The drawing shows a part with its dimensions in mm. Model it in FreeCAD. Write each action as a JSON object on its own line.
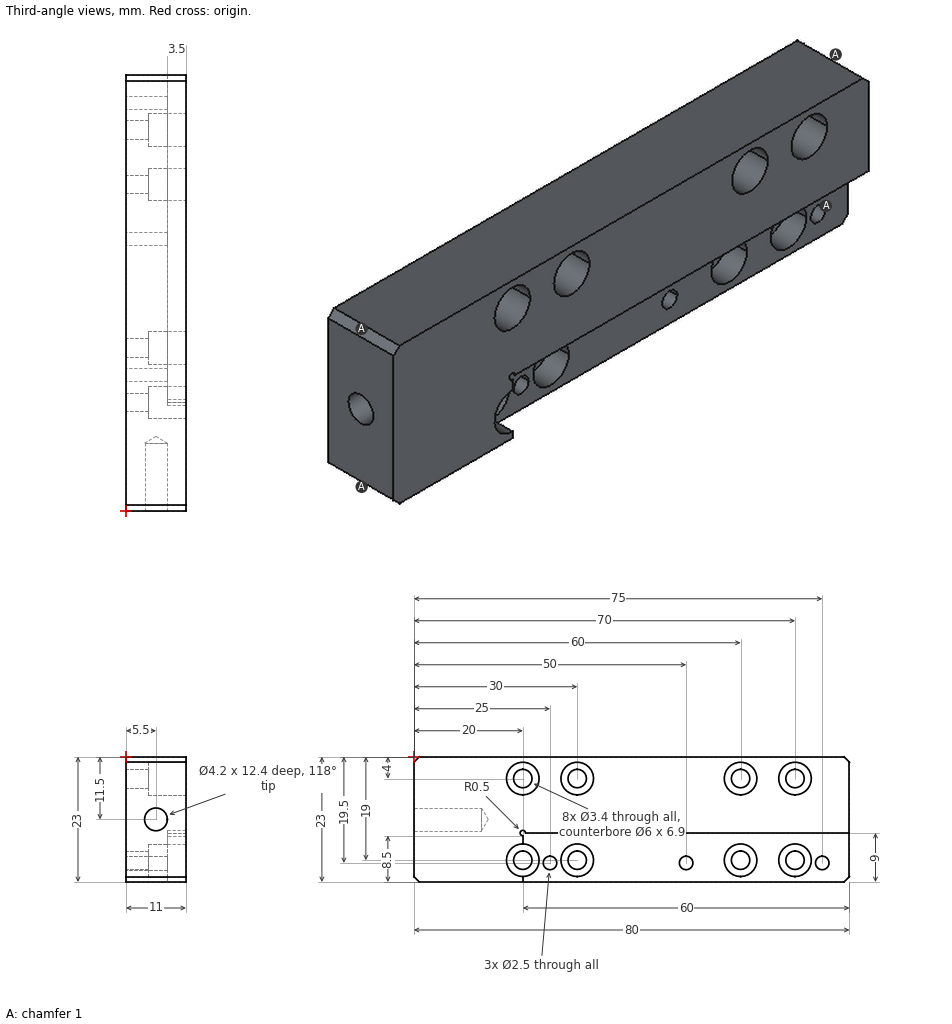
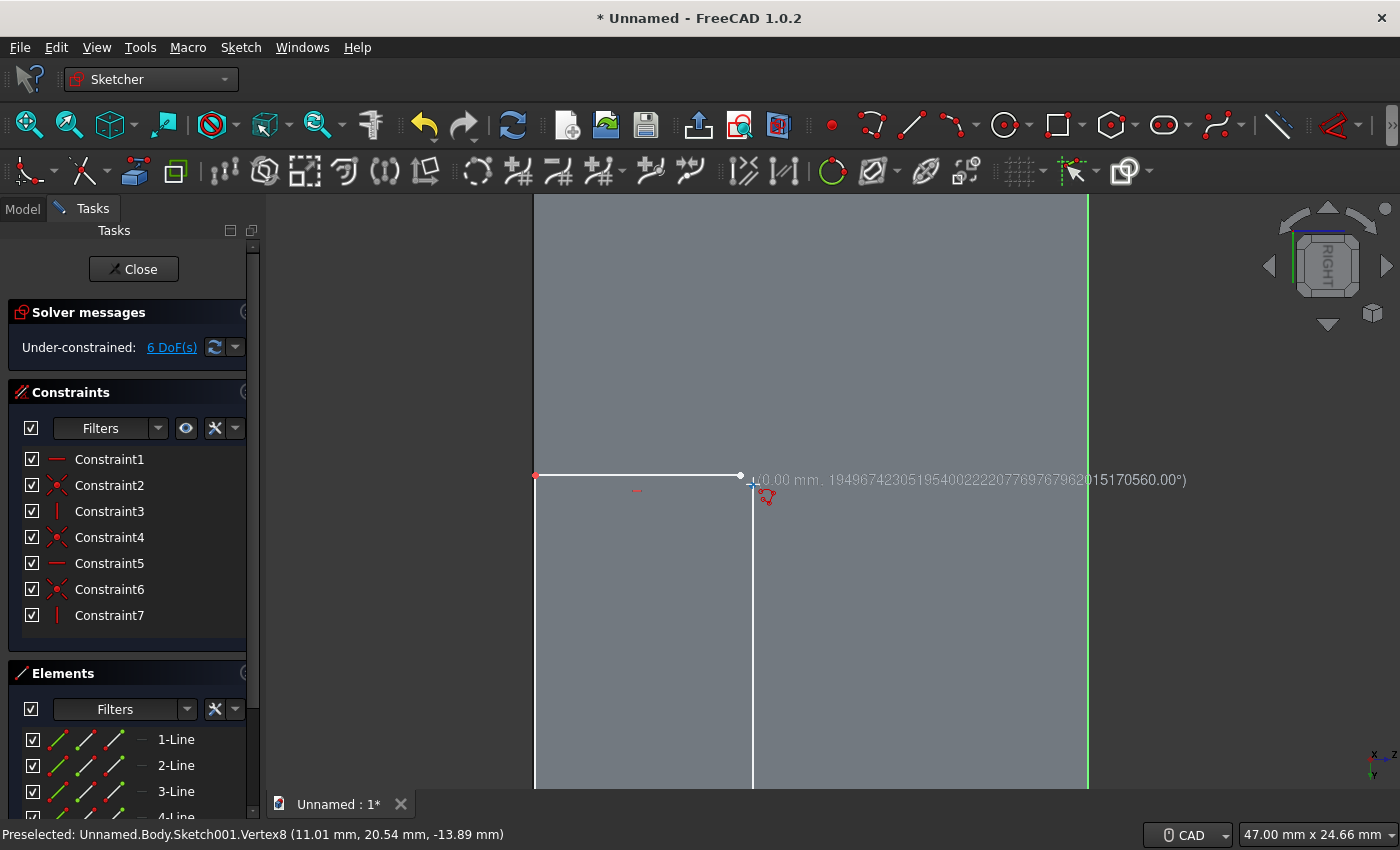
{"action": "left_click", "coordinate": [952, 126]}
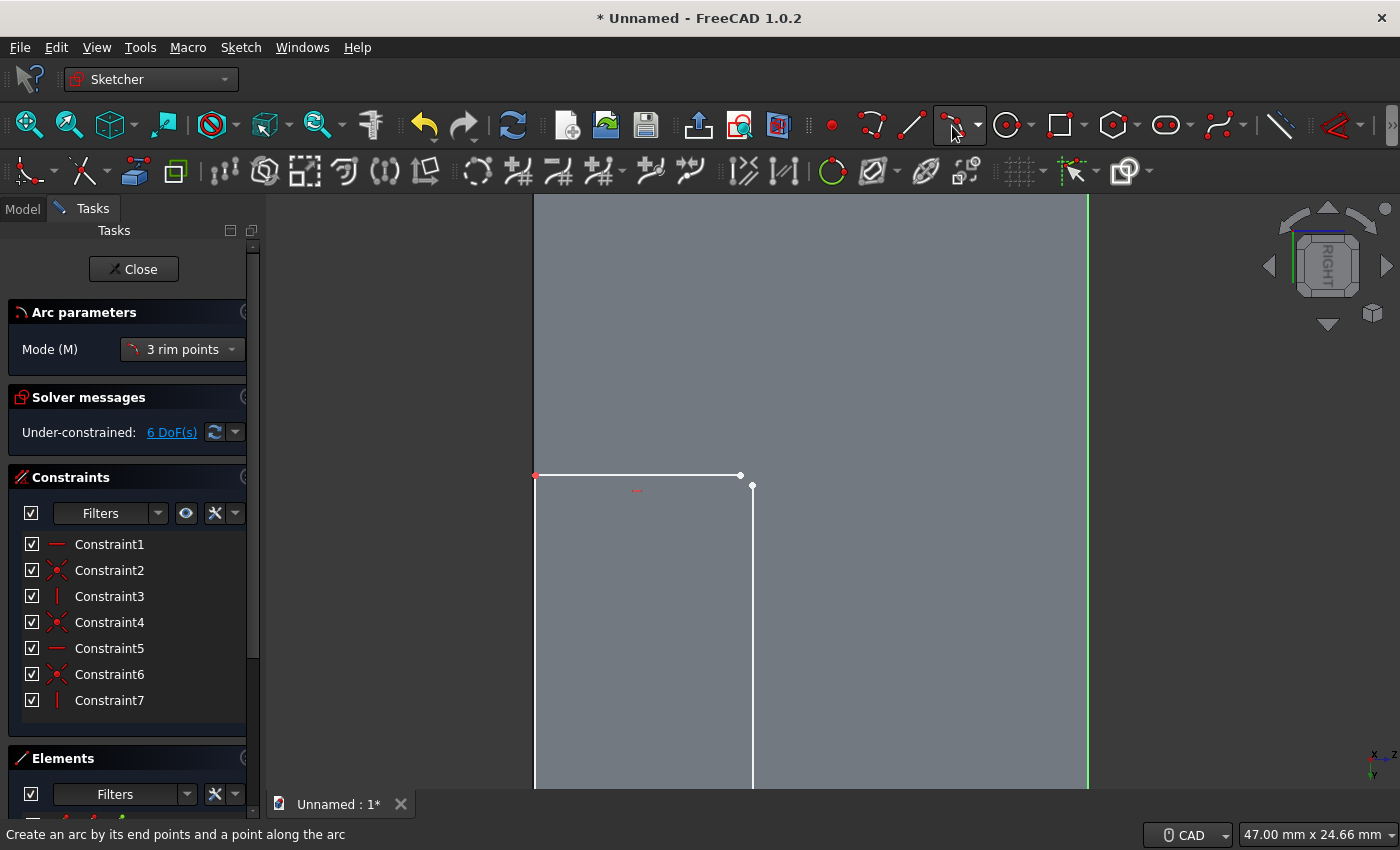
{"action": "left_click", "coordinate": [753, 485]}
{"action": "left_click", "coordinate": [741, 475]}
{"action": "left_click", "coordinate": [759, 464]}
{"action": "key", "text": "Escape"}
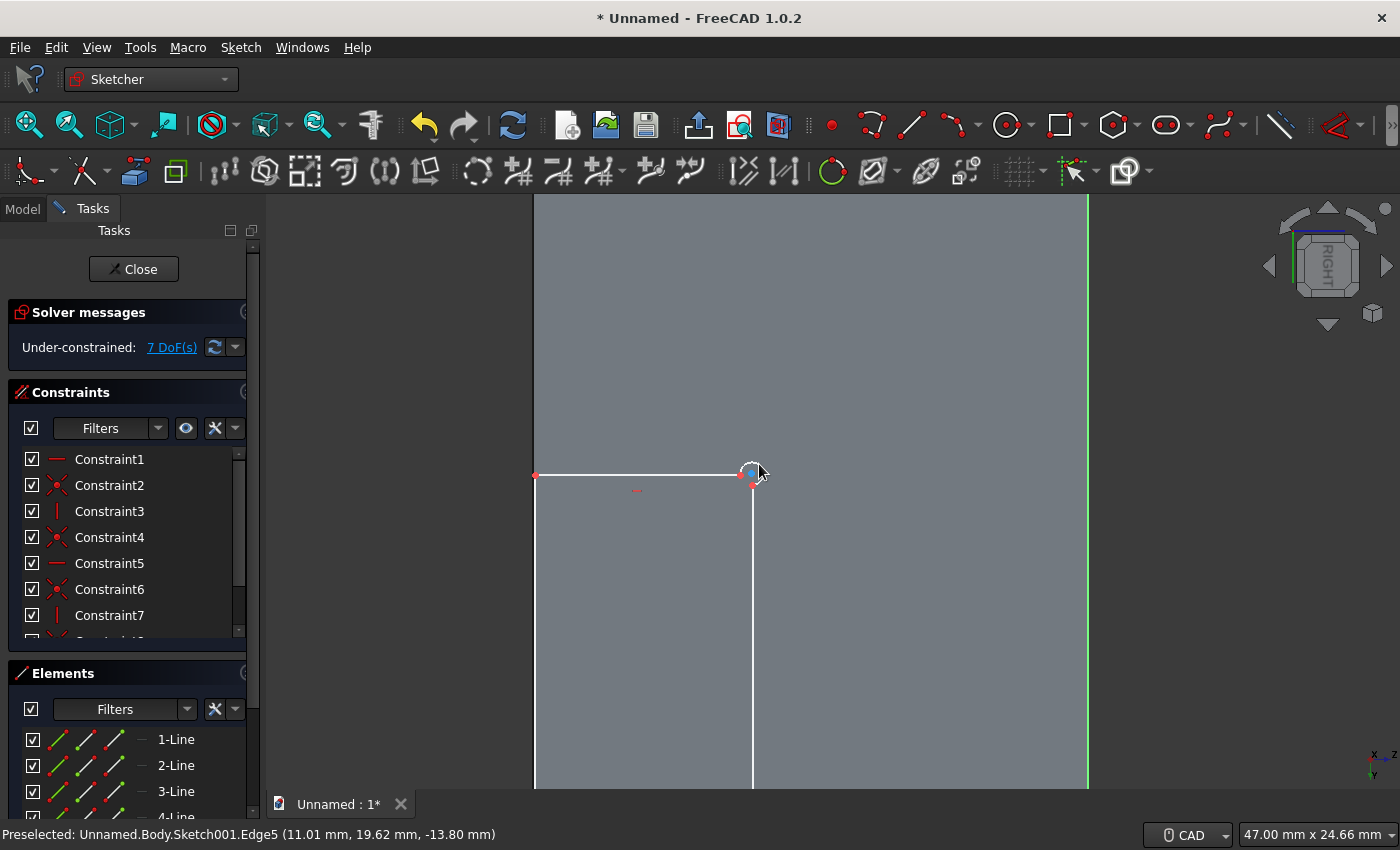
{"action": "left_click", "coordinate": [1336, 126]}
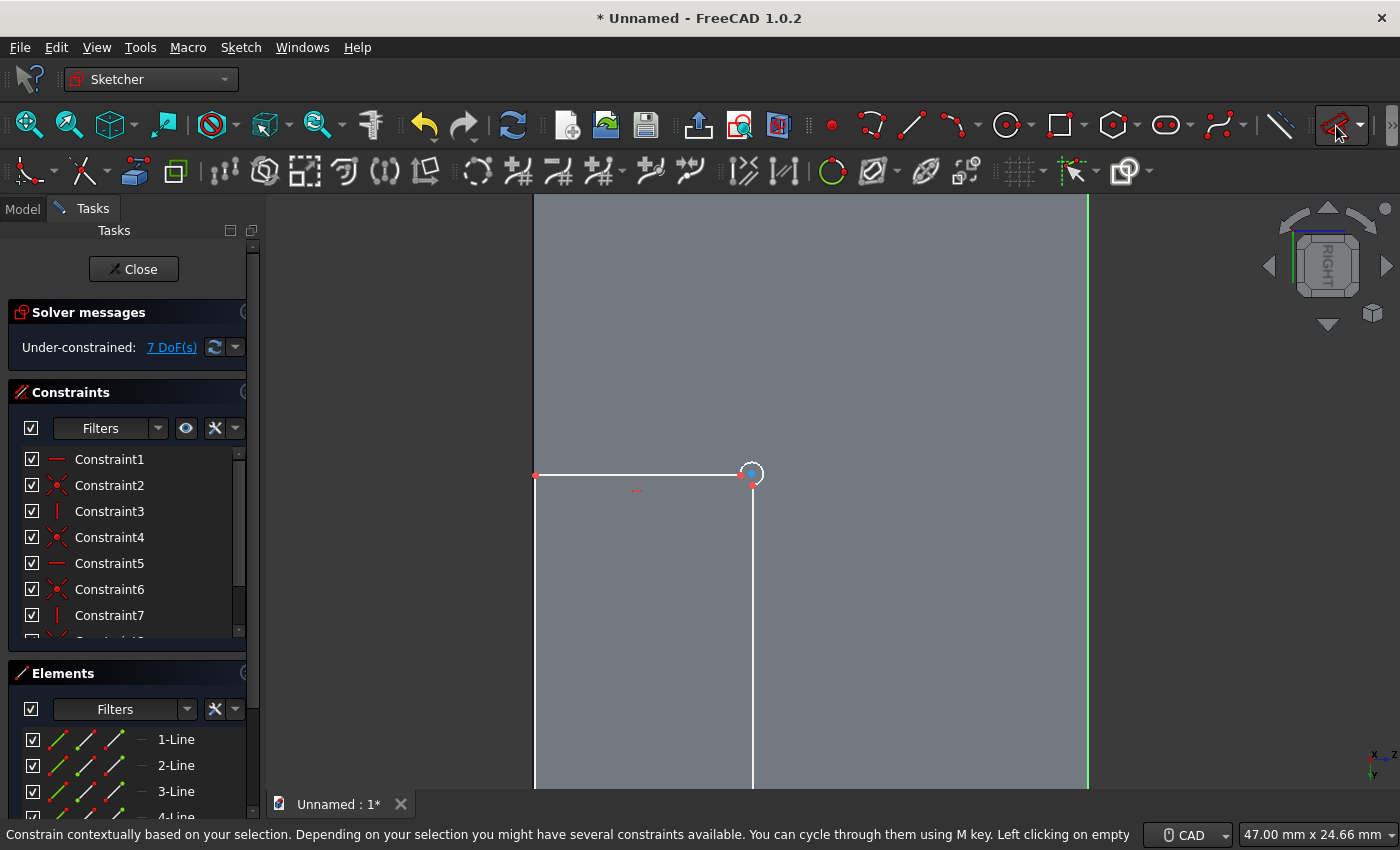
{"action": "scroll", "coordinate": [763, 474], "scroll_direction": "up", "scroll_amount": 6}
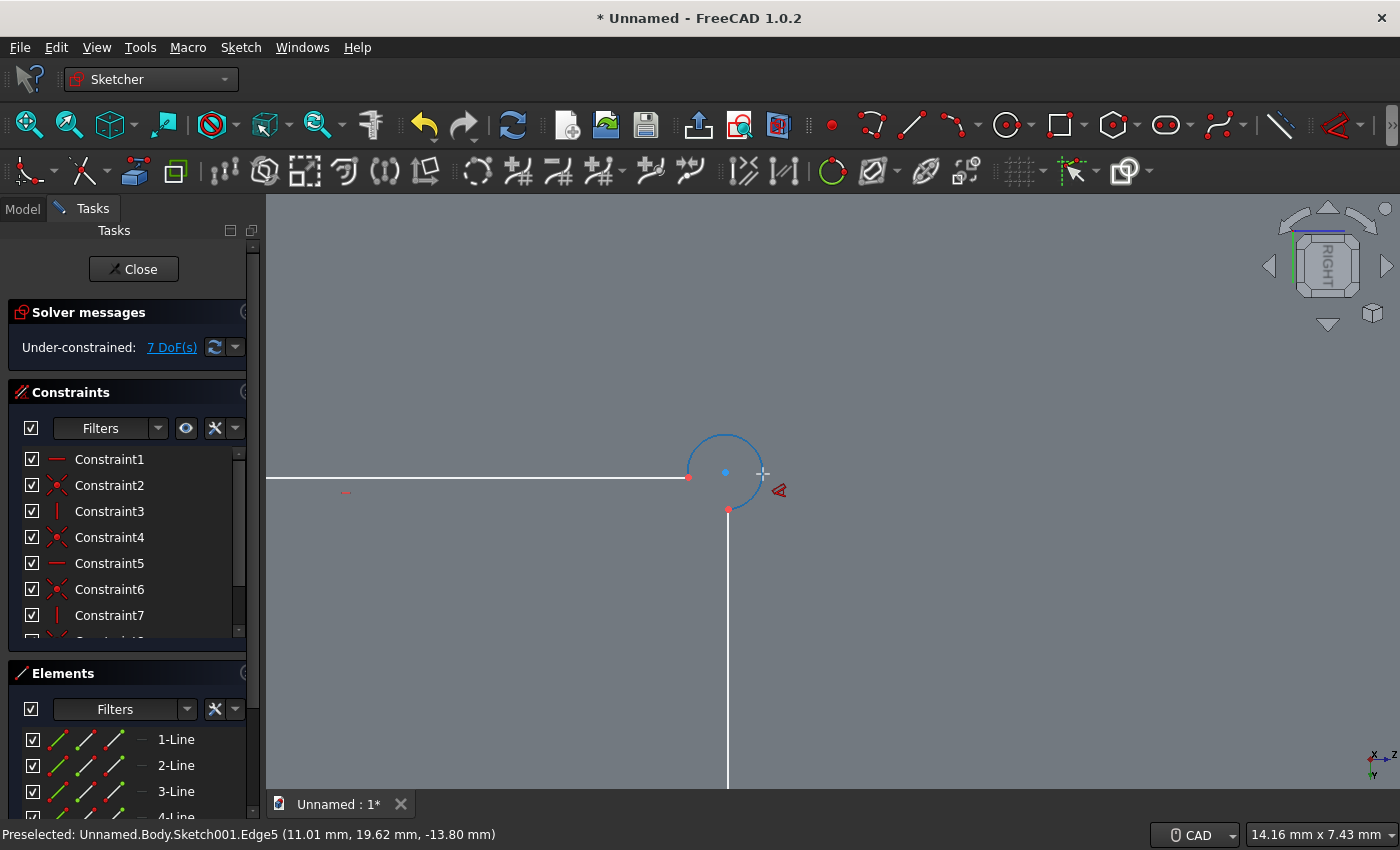
{"action": "left_click", "coordinate": [762, 474]}
{"action": "left_click", "coordinate": [794, 476]}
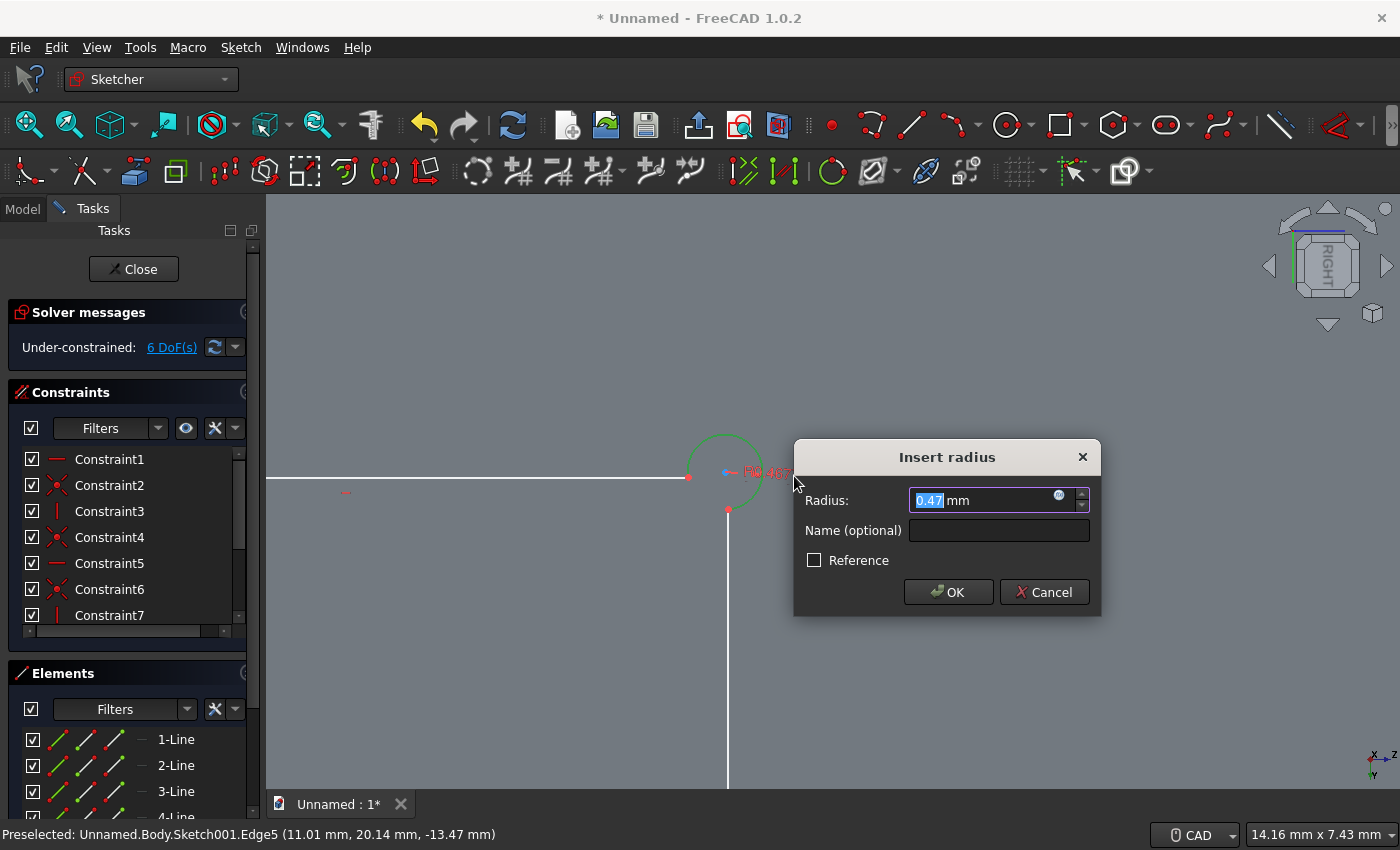
{"action": "type", "text": "0.5"}
{"action": "key", "text": "Return"}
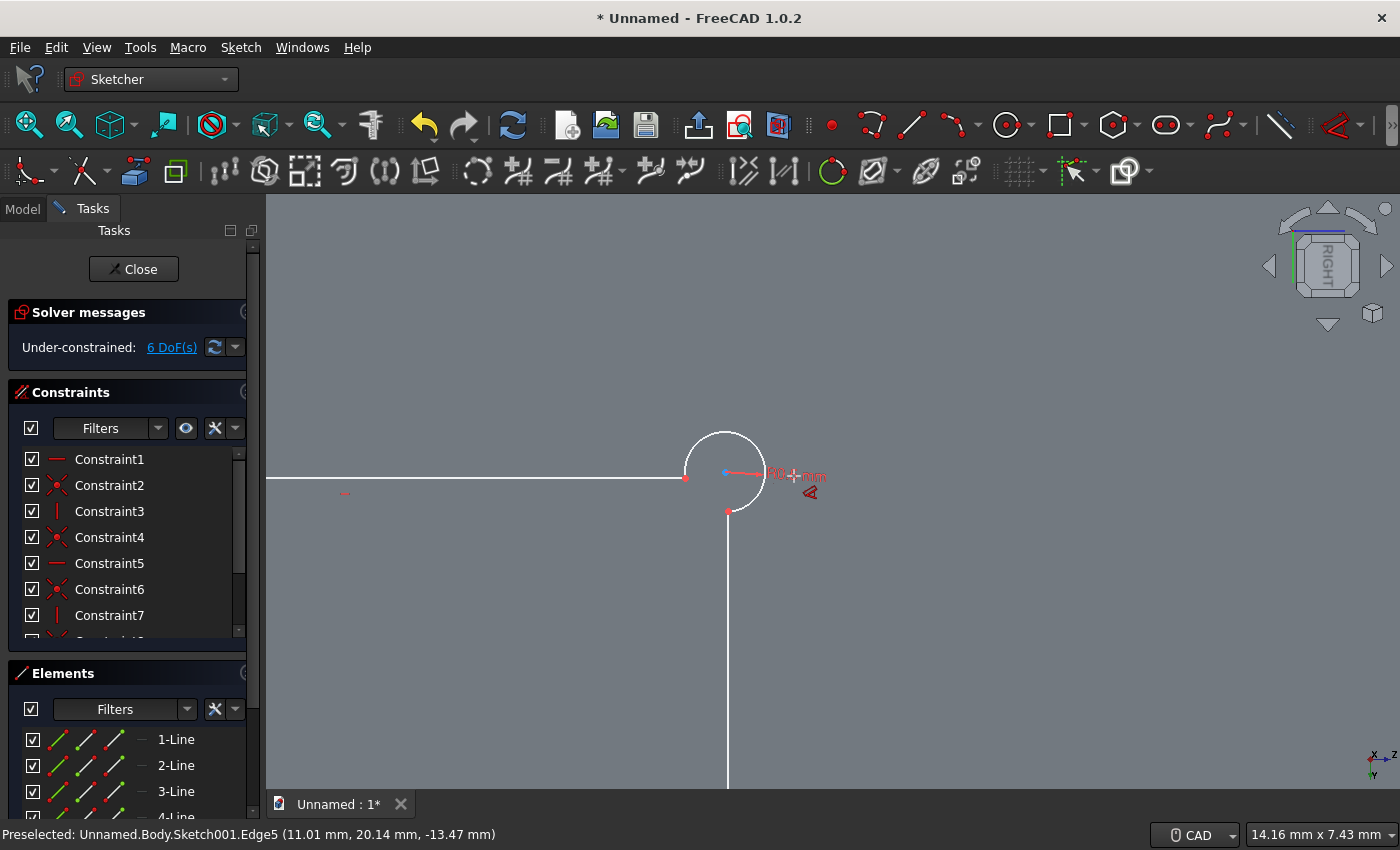
{"action": "scroll", "coordinate": [754, 389], "scroll_direction": "down", "scroll_amount": 14}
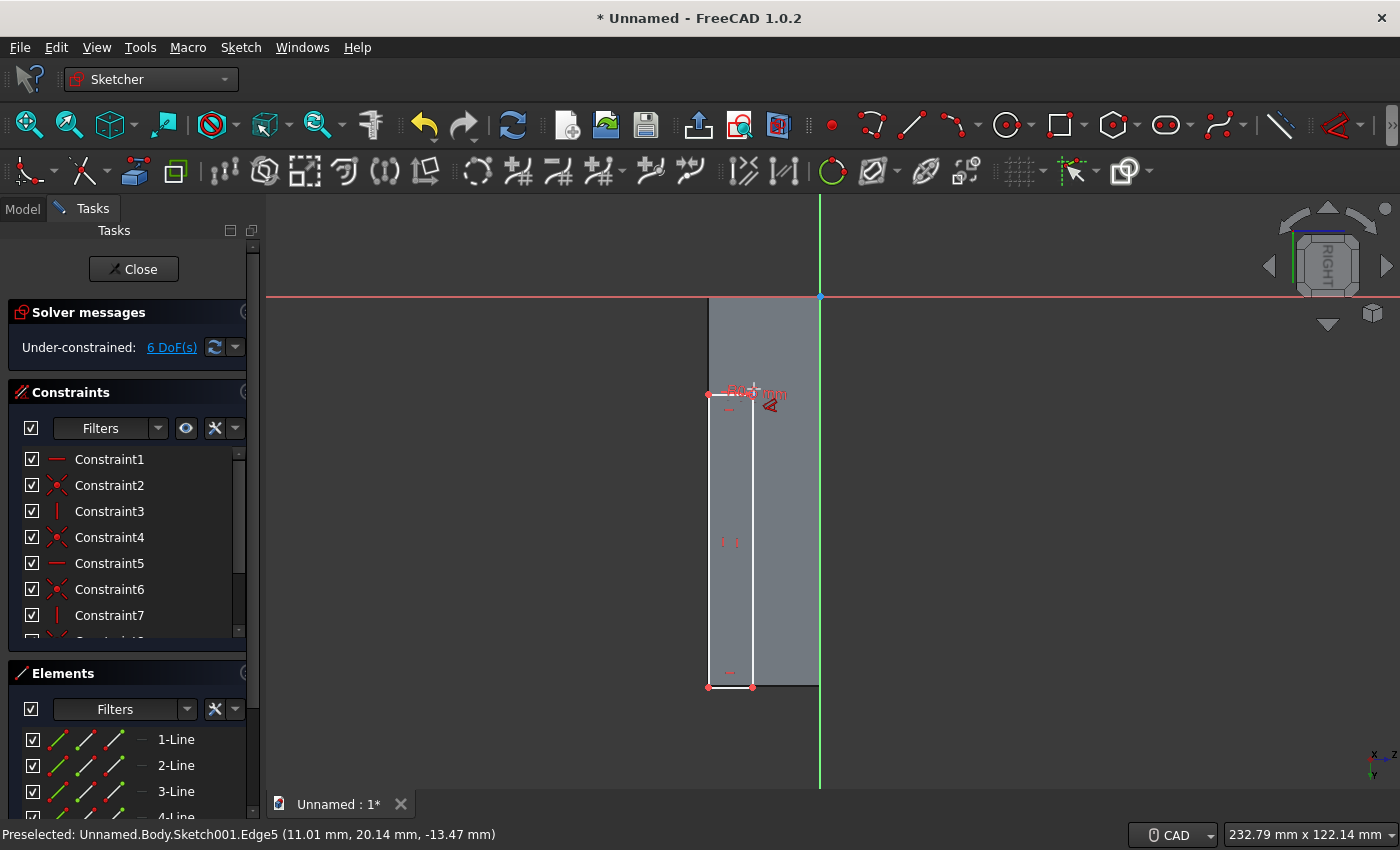
{"action": "left_click", "coordinate": [722, 688]}
{"action": "left_click", "coordinate": [731, 722]}